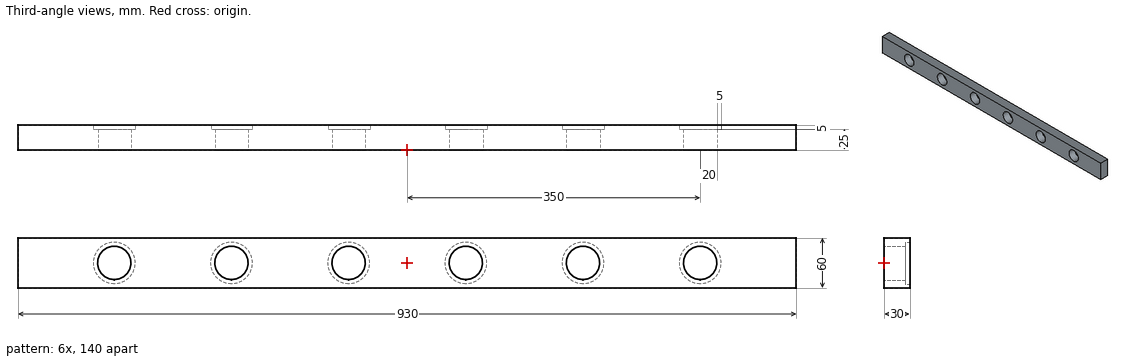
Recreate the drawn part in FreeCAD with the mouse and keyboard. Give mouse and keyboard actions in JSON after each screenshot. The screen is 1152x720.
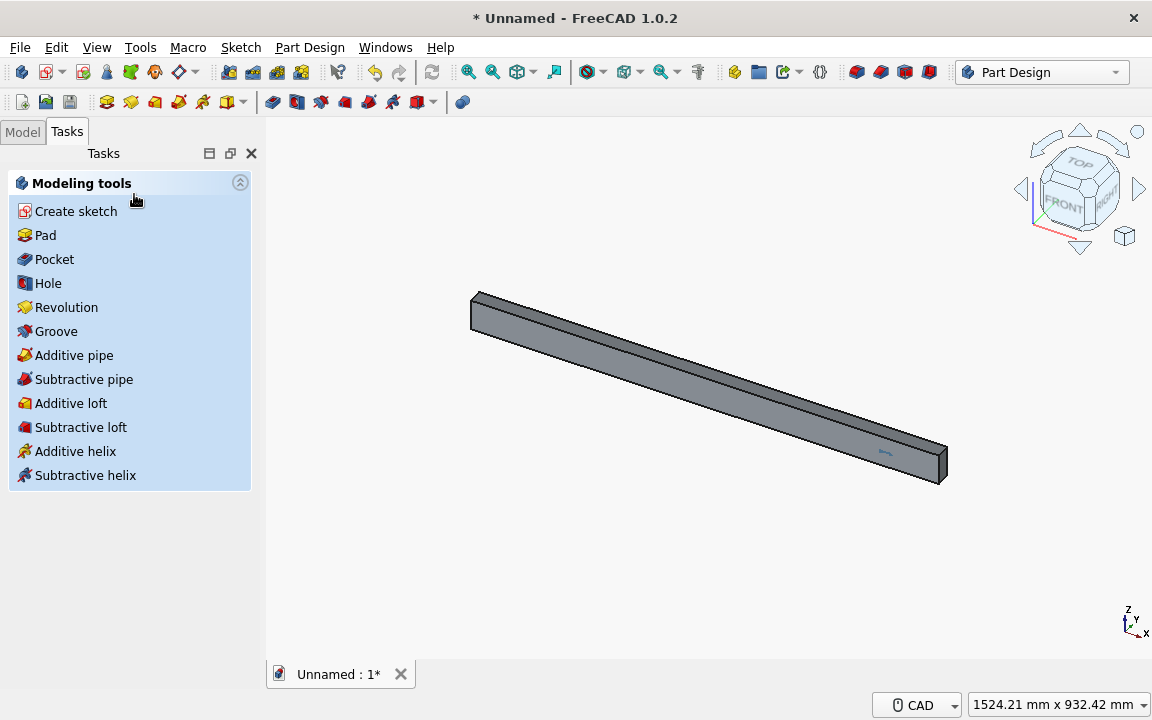
{"action": "left_click", "coordinate": [322, 102]}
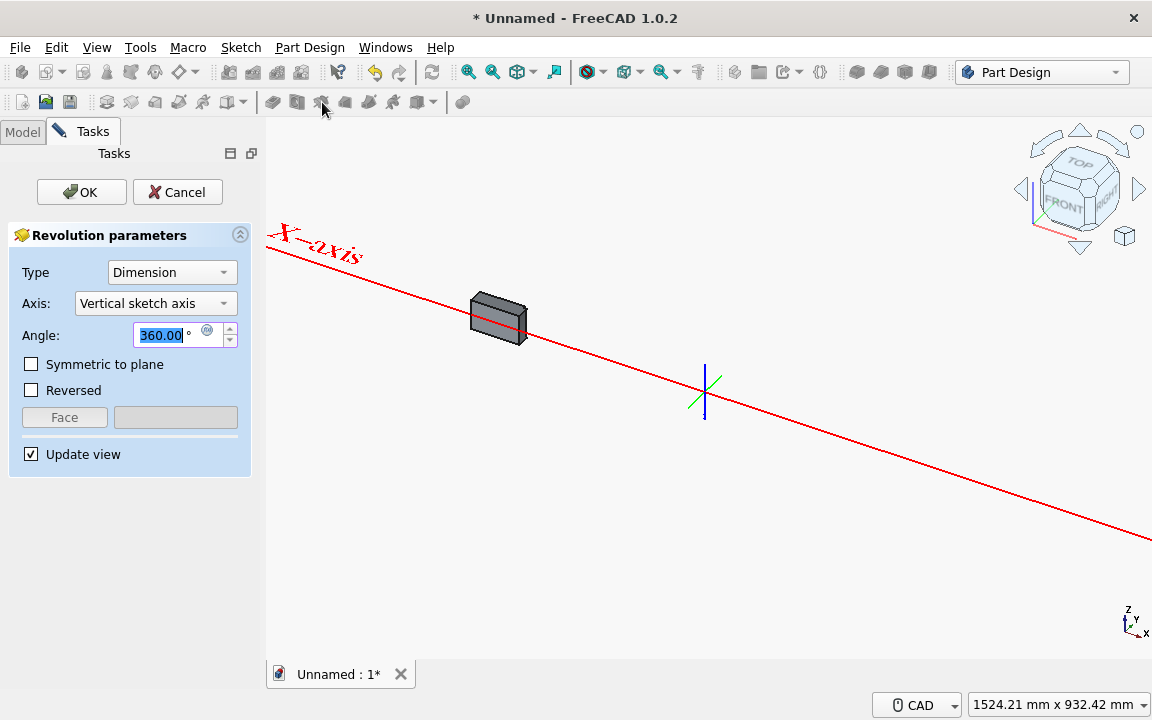
{"action": "left_click", "coordinate": [156, 304]}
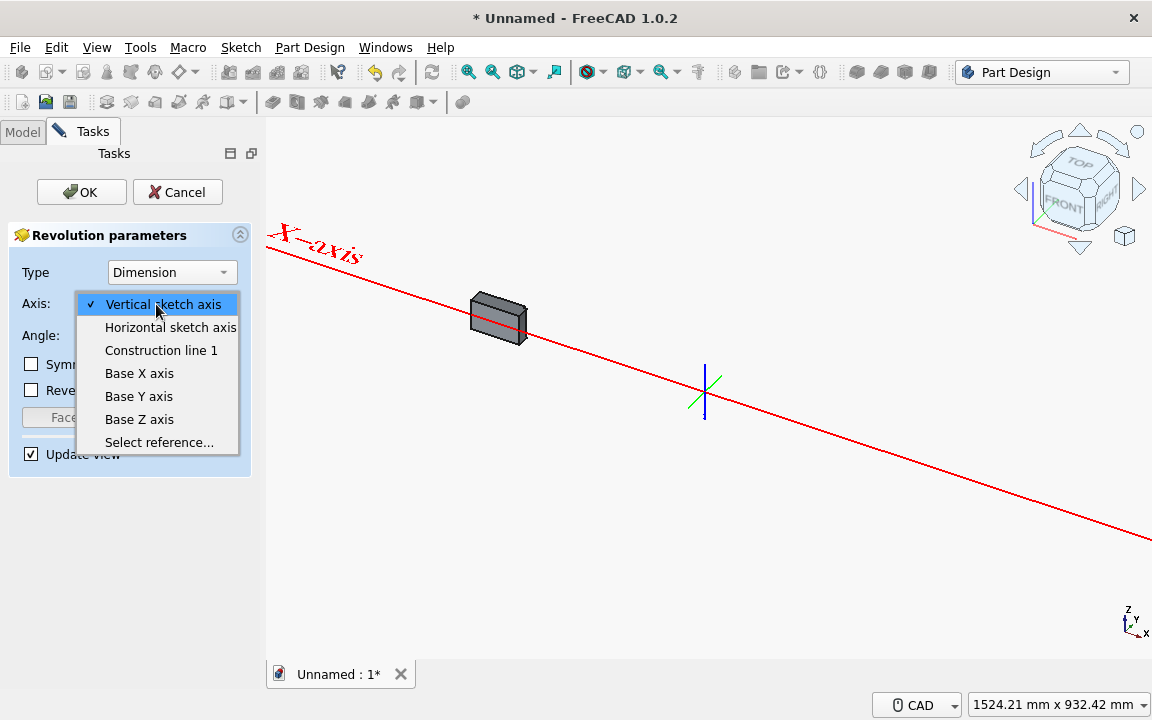
{"action": "left_click", "coordinate": [156, 350]}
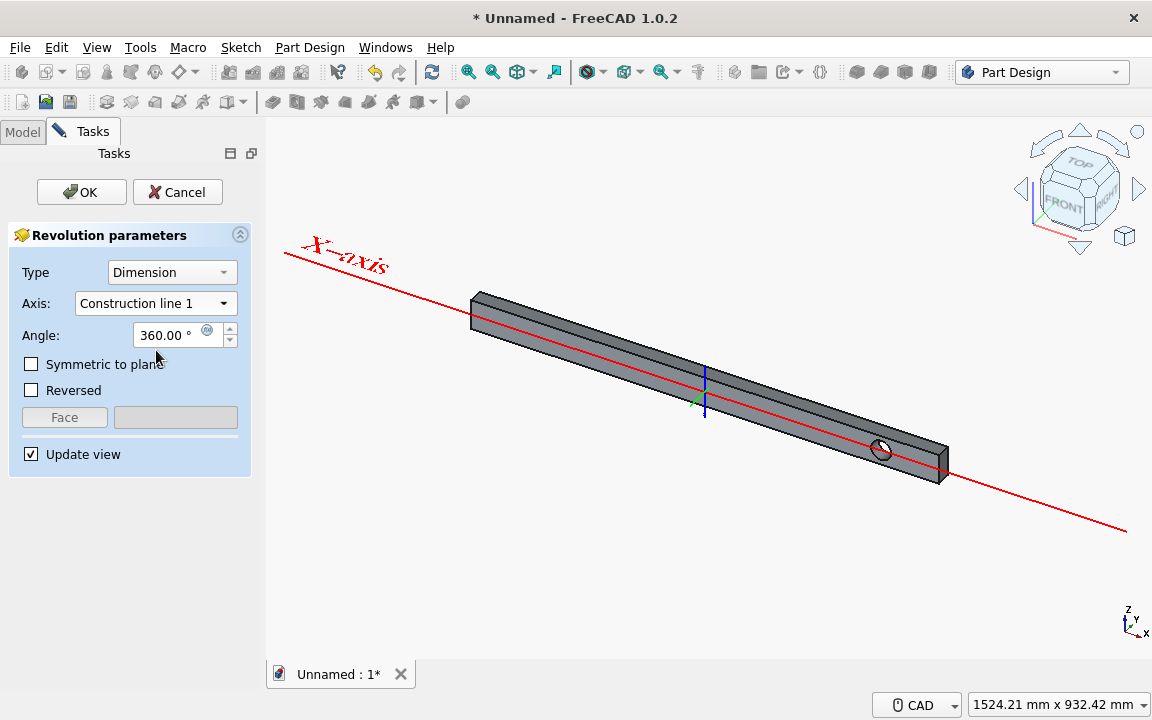
{"action": "left_click", "coordinate": [82, 192]}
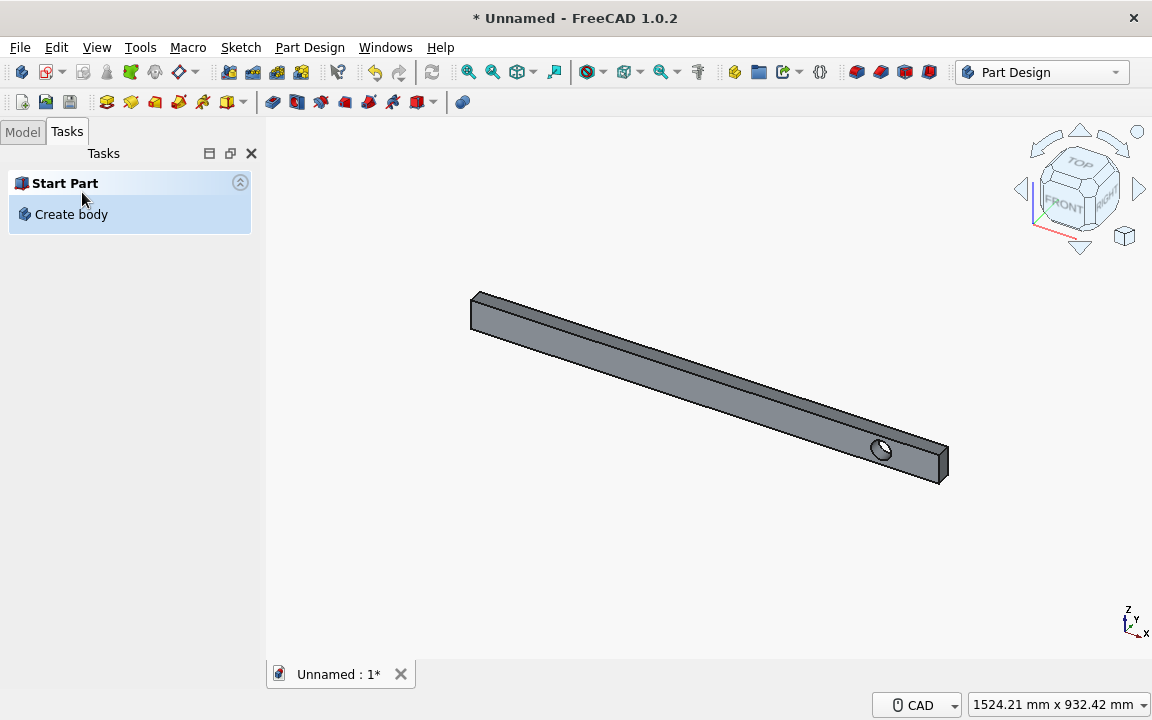
{"action": "left_click", "coordinate": [23, 131]}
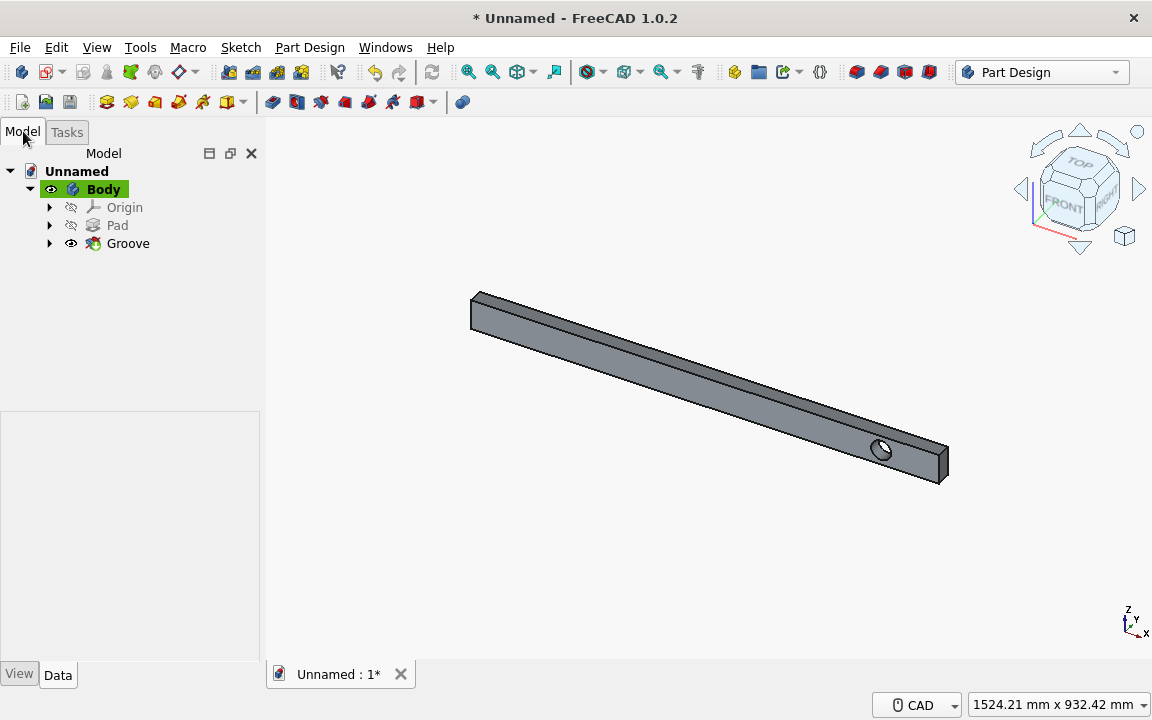
{"action": "left_click", "coordinate": [116, 243]}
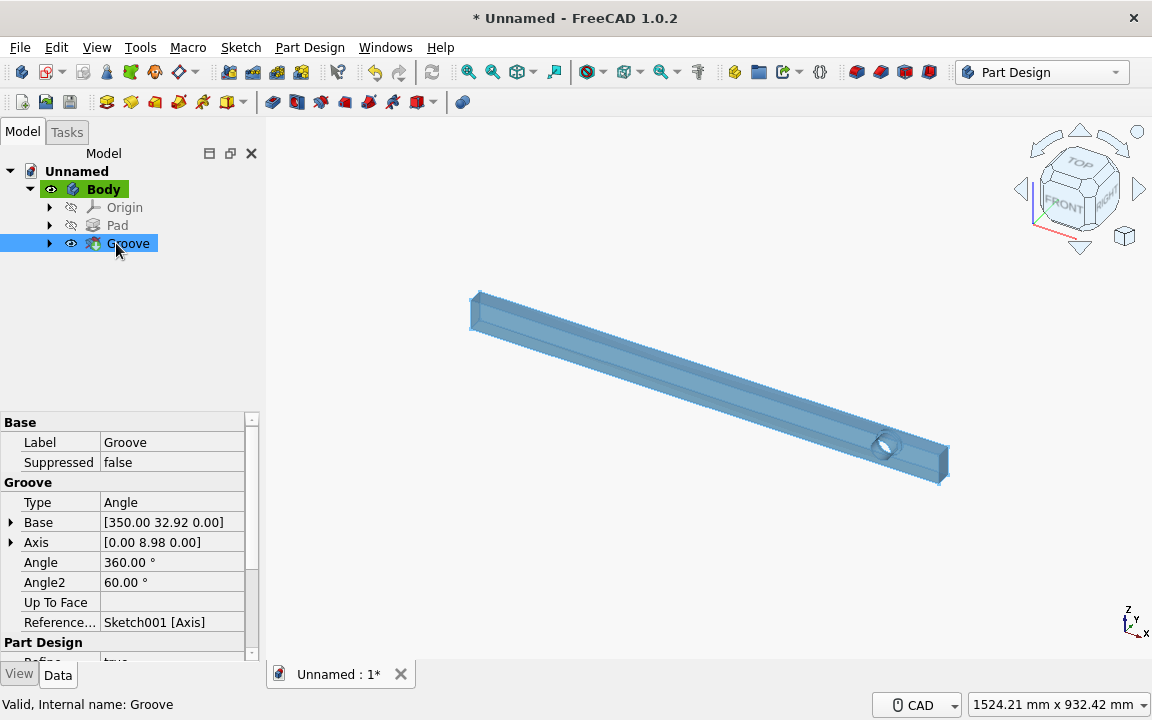
{"action": "left_click", "coordinate": [254, 72]}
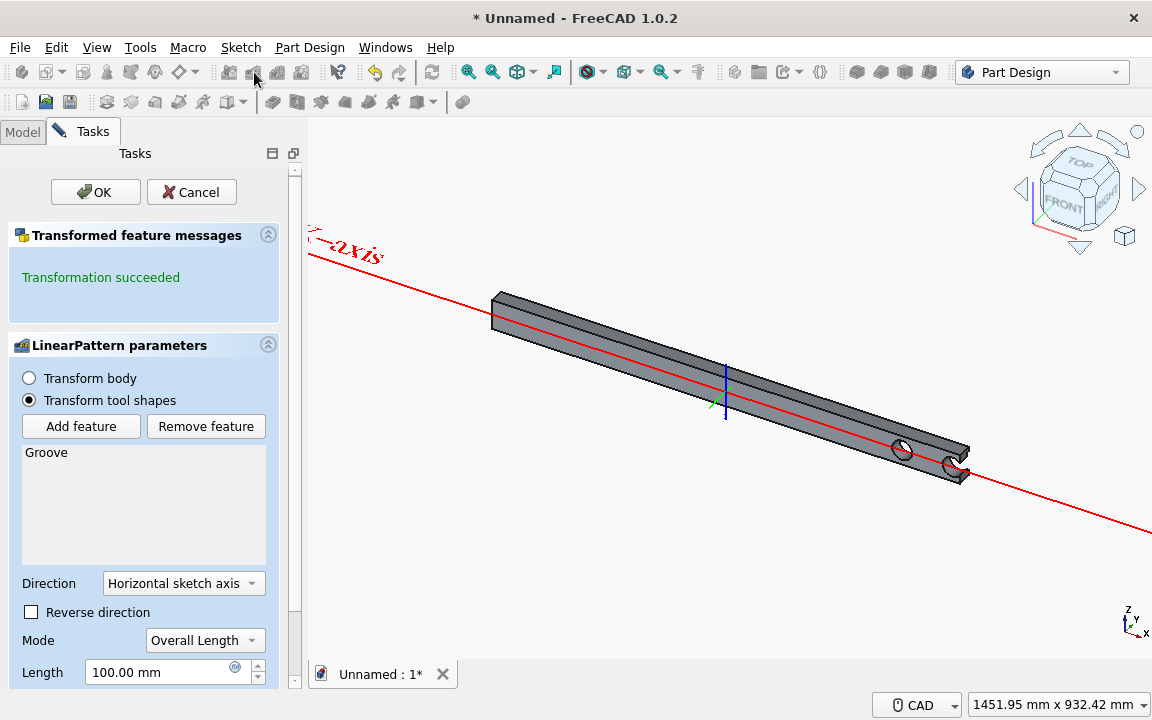
{"action": "left_click", "coordinate": [184, 584]}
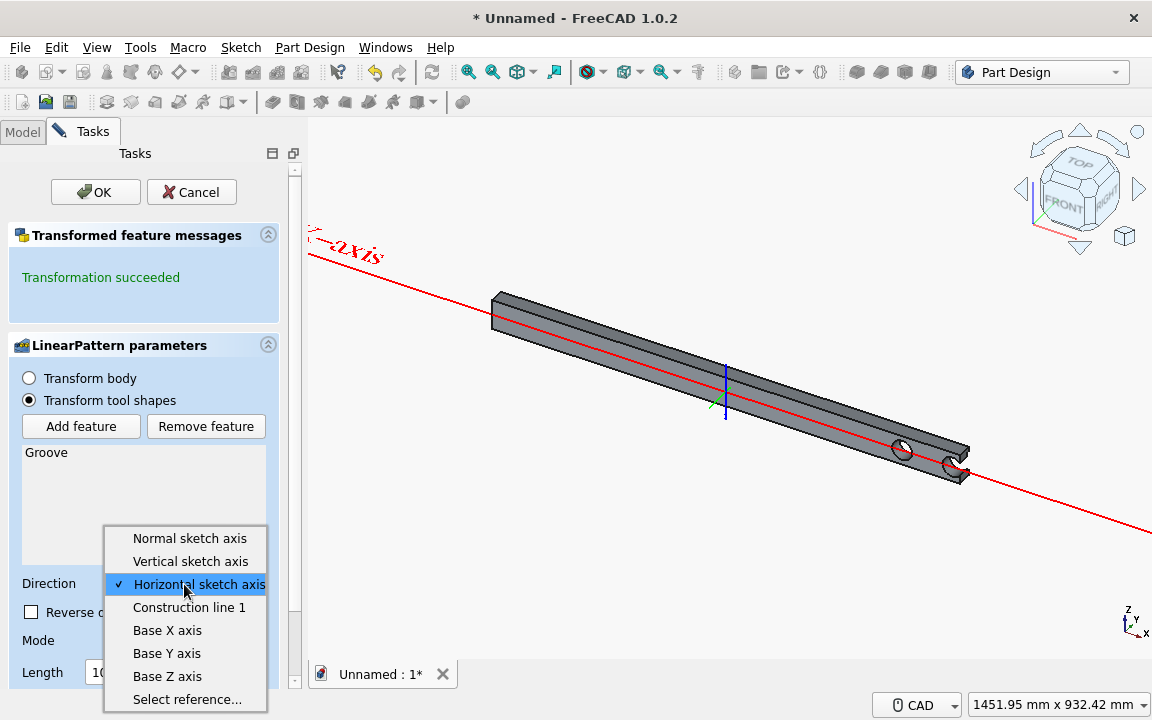
{"action": "left_click", "coordinate": [184, 630]}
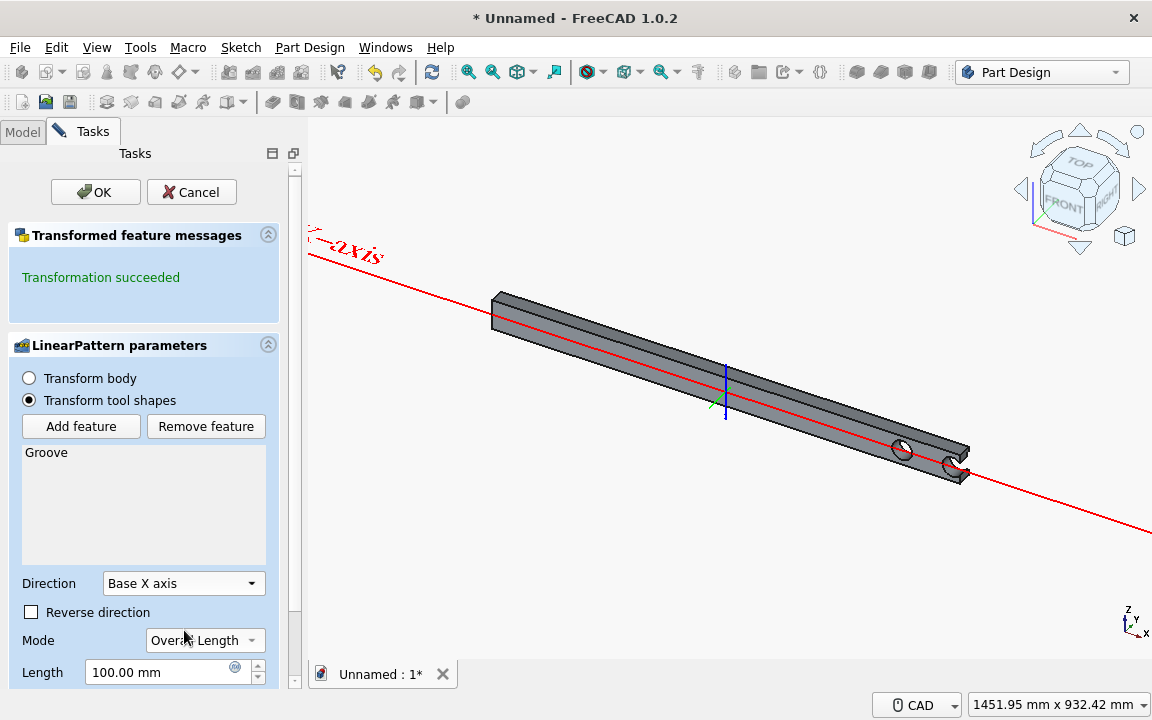
{"action": "left_click", "coordinate": [206, 640]}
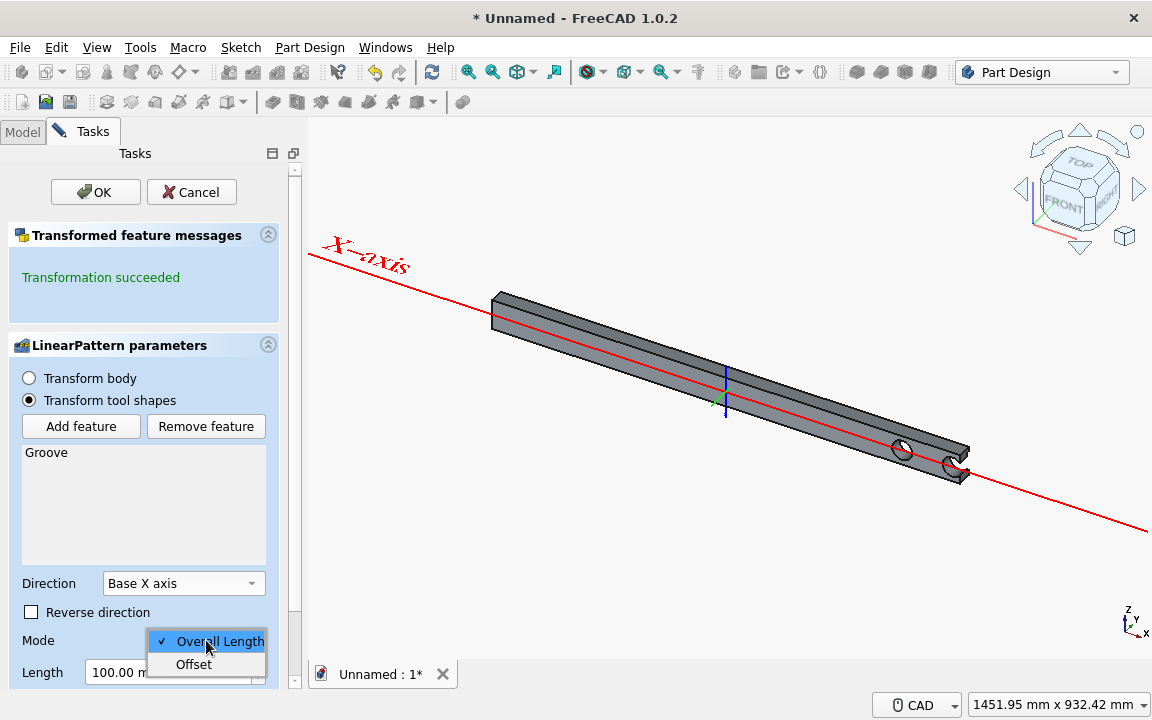
{"action": "left_click", "coordinate": [206, 664]}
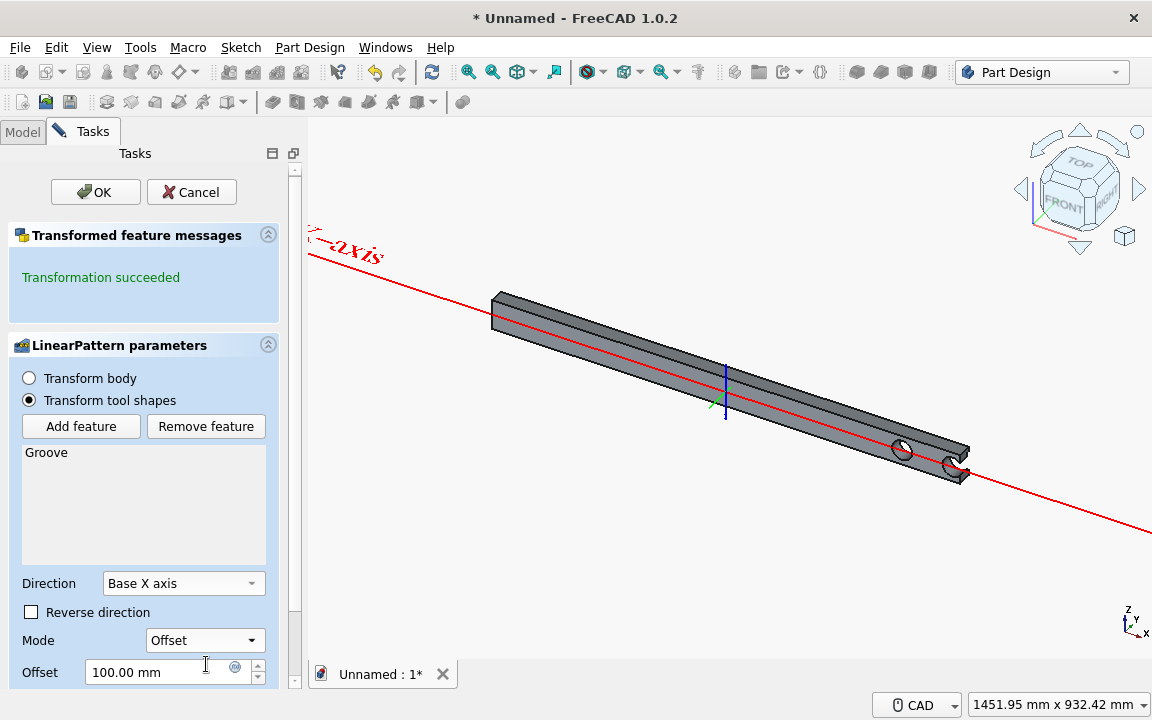
{"action": "triple_click", "coordinate": [168, 672]}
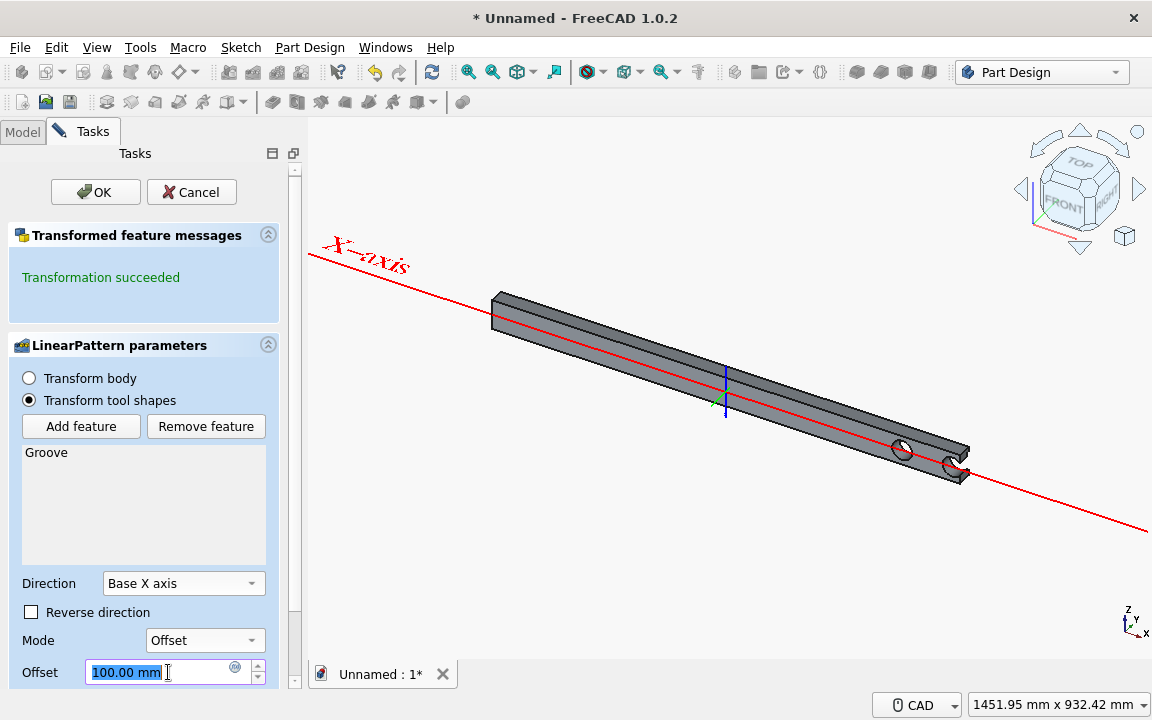
{"action": "type", "text": "140"}
{"action": "key", "text": "Tab"}